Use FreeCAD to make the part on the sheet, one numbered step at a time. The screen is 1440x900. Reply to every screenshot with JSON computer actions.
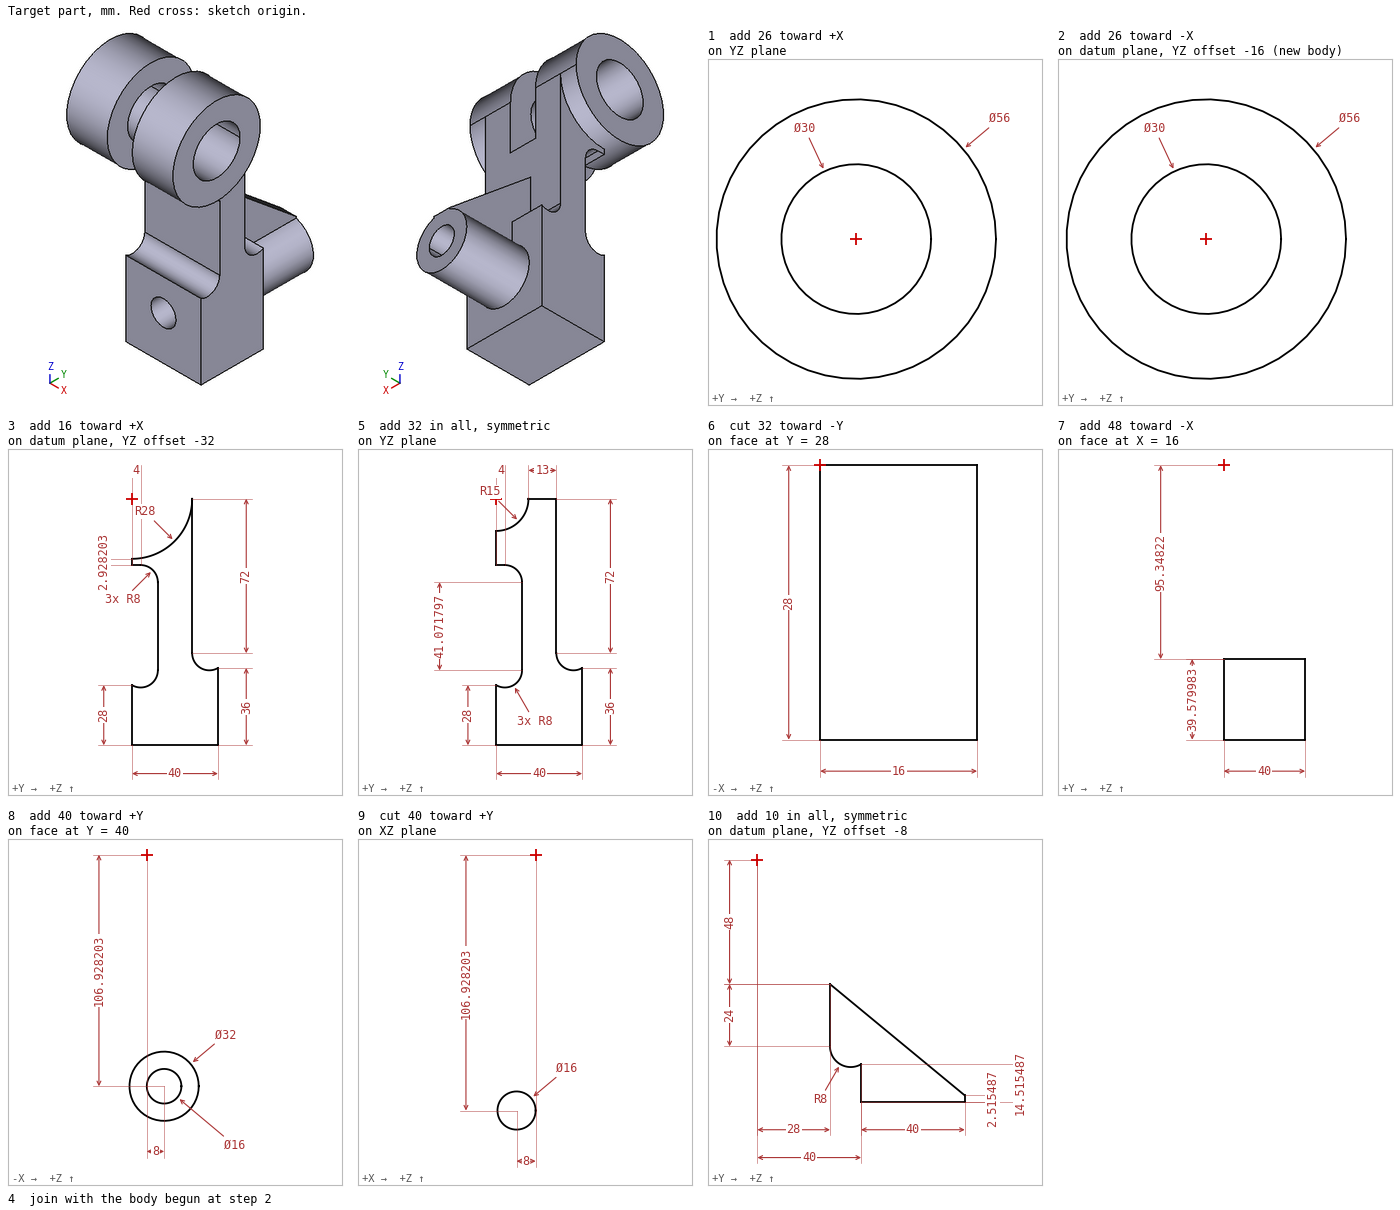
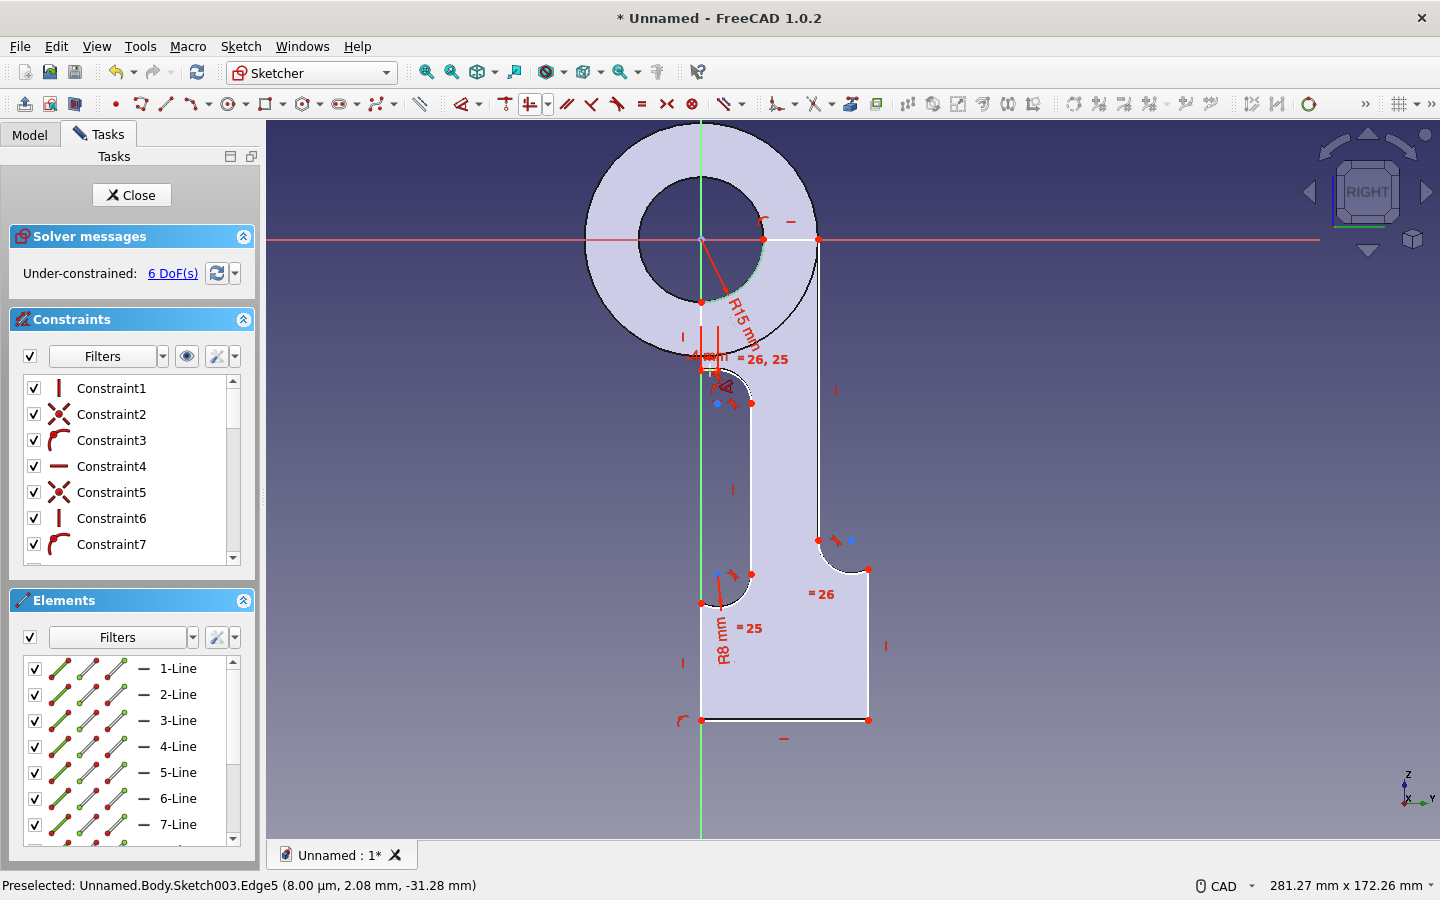
{"action": "left_click", "coordinate": [868, 615]}
{"action": "left_click", "coordinate": [902, 645]}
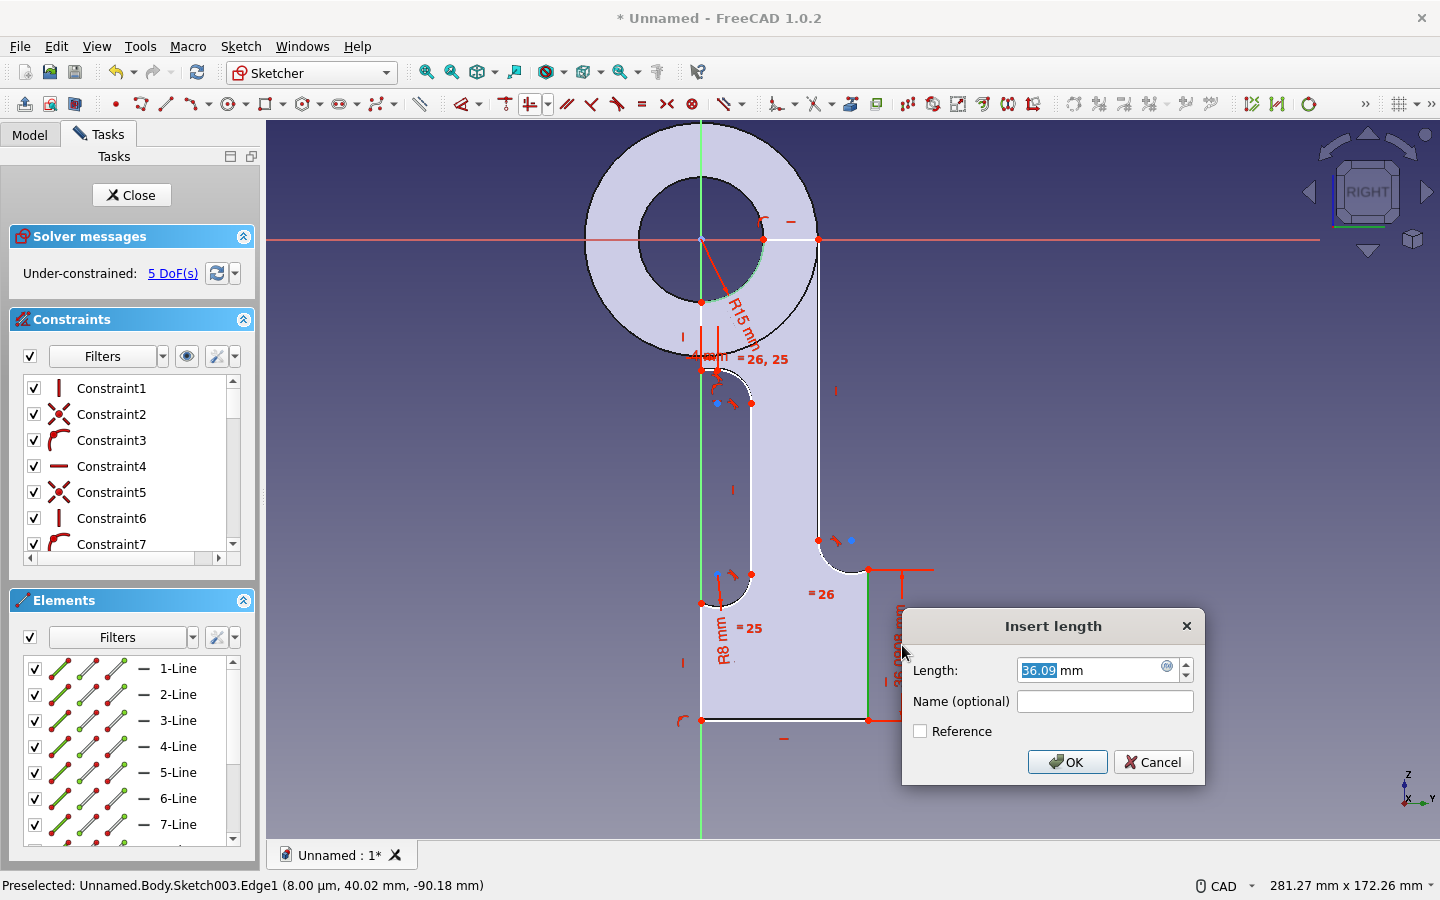
{"action": "type", "text": "36"}
{"action": "key", "text": "Return"}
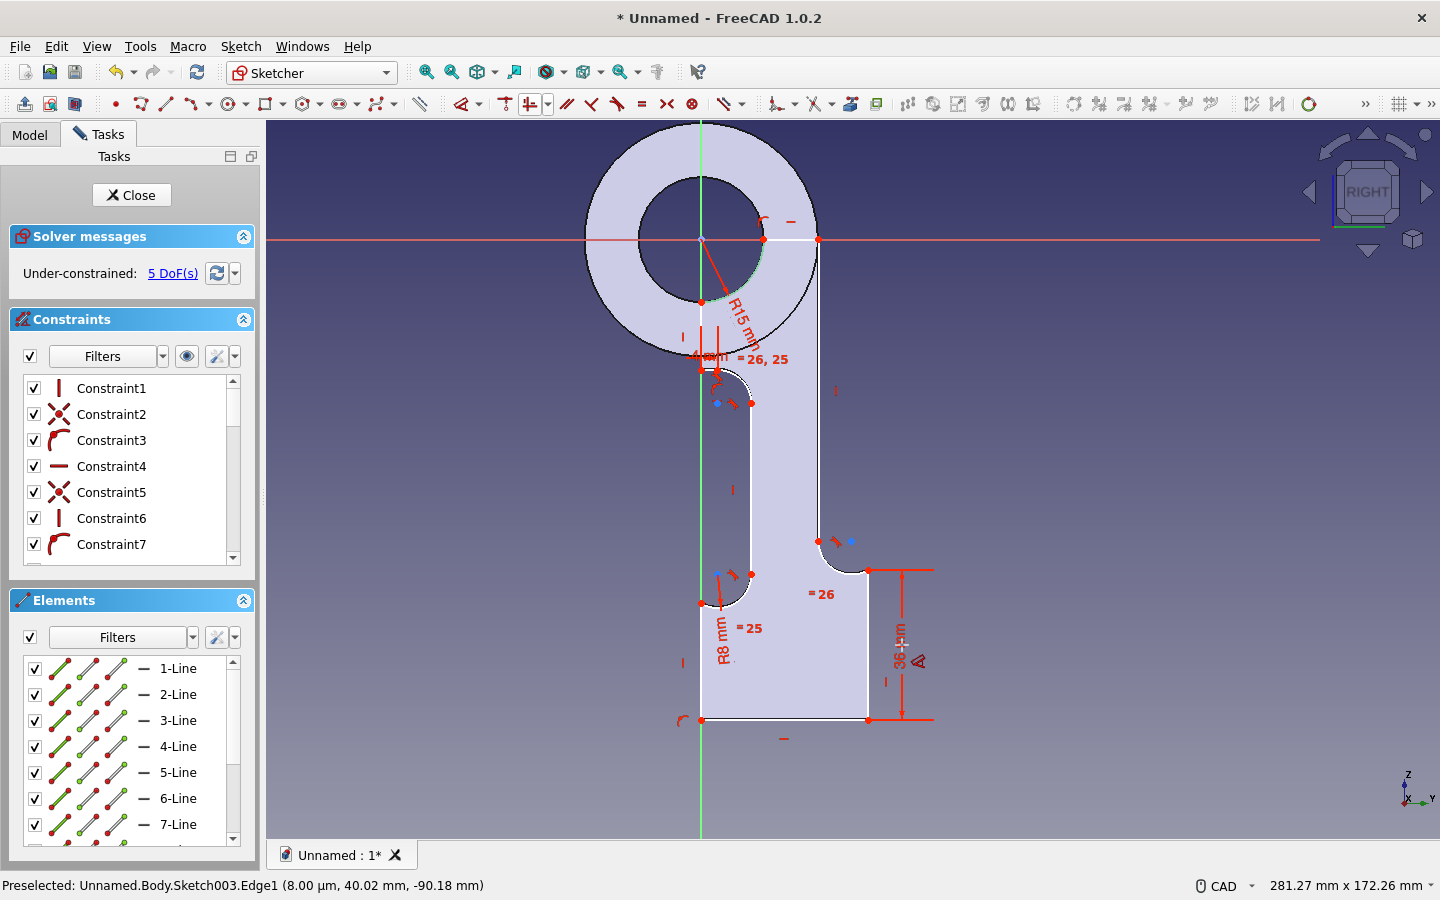
{"action": "left_click", "coordinate": [818, 720]}
{"action": "left_click", "coordinate": [785, 754]}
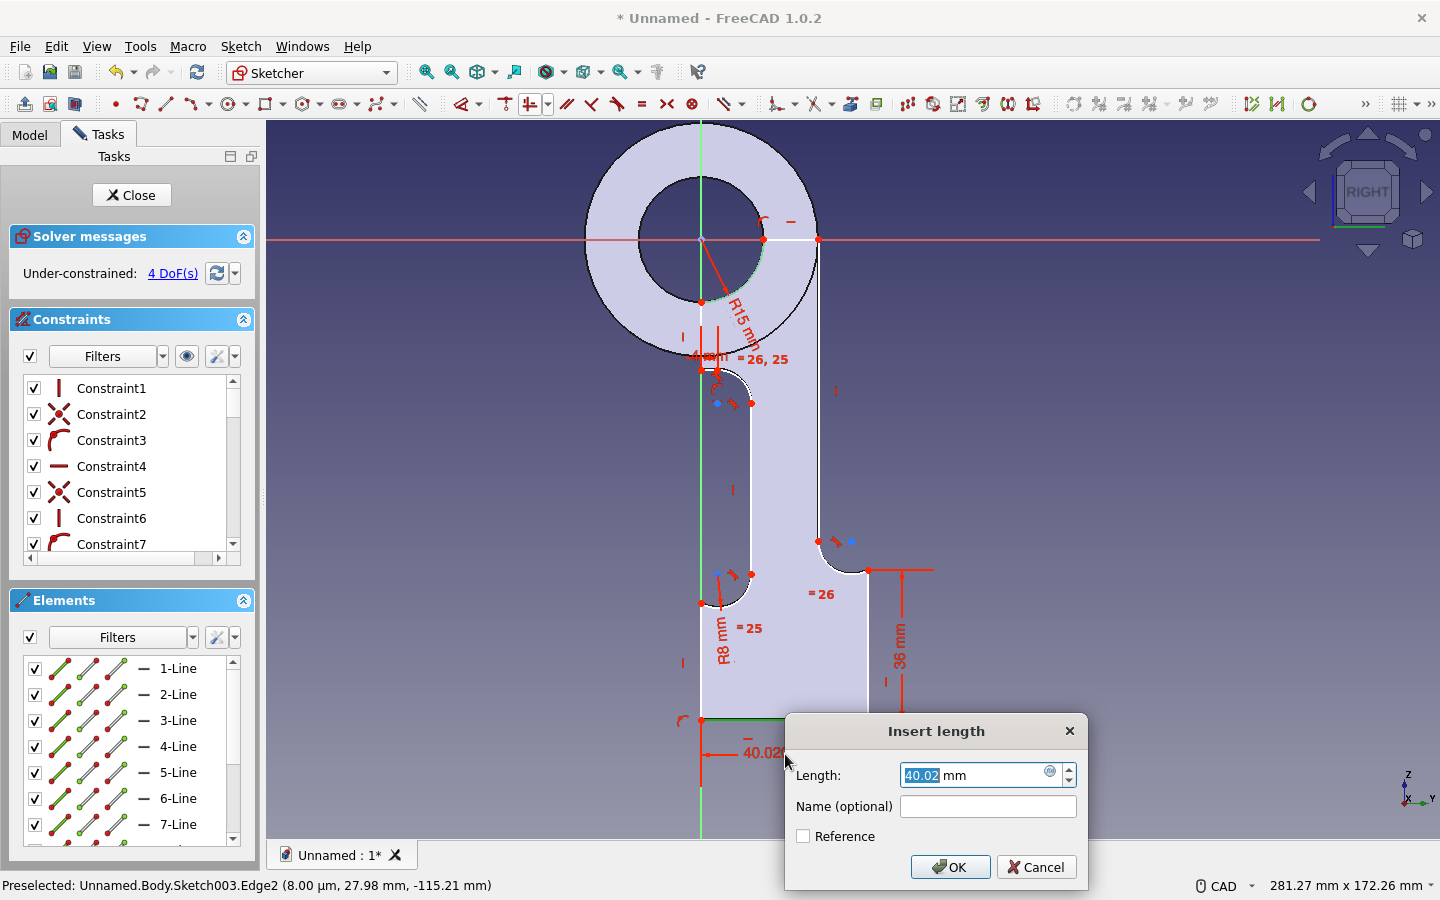
{"action": "type", "text": "40"}
{"action": "key", "text": "Return"}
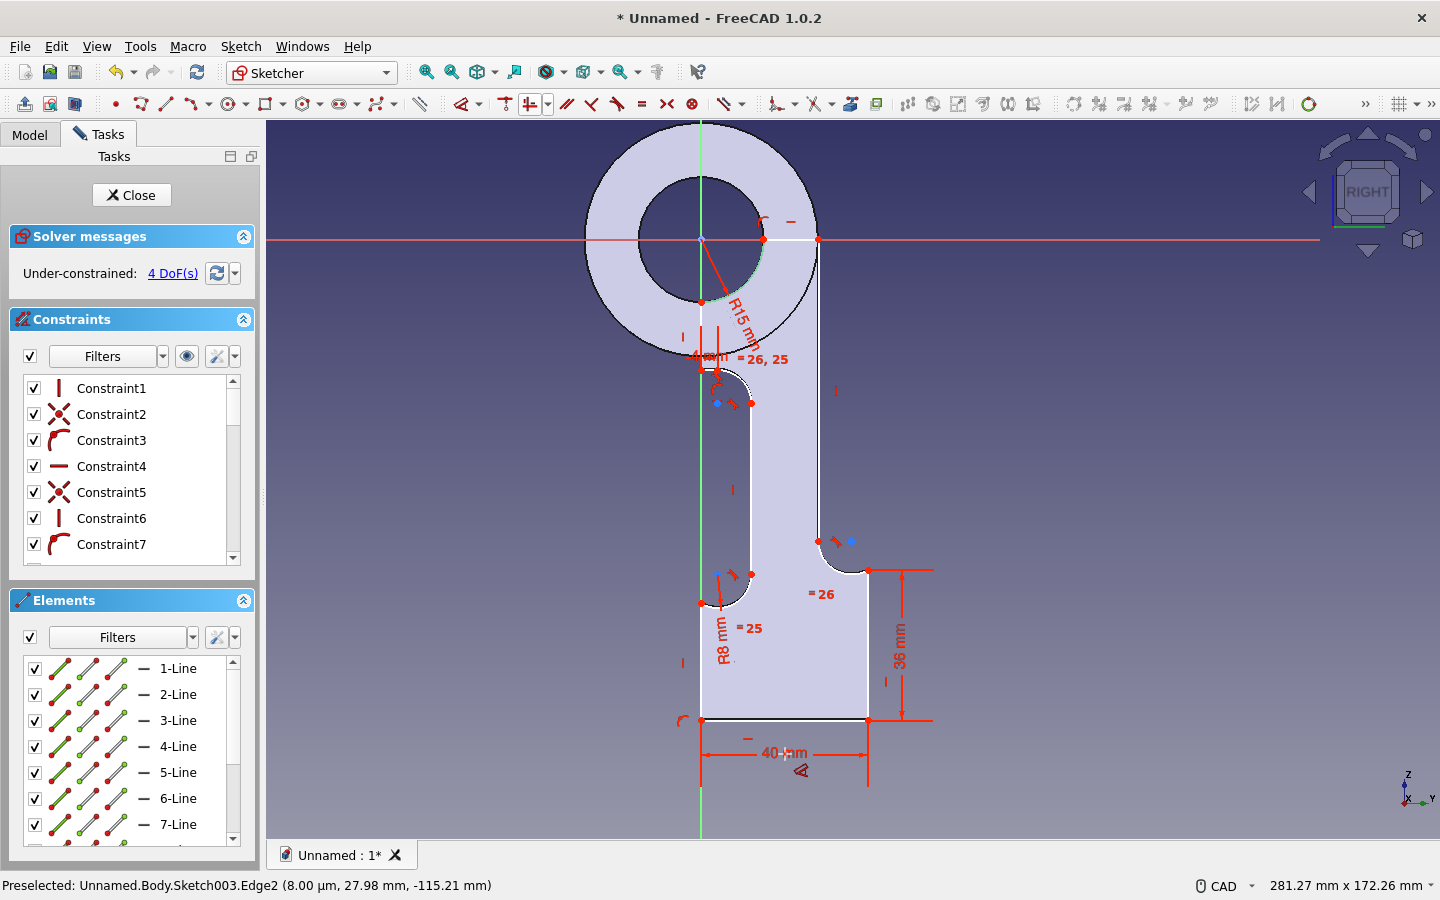
{"action": "left_click", "coordinate": [701, 685]}
{"action": "left_click", "coordinate": [667, 662]}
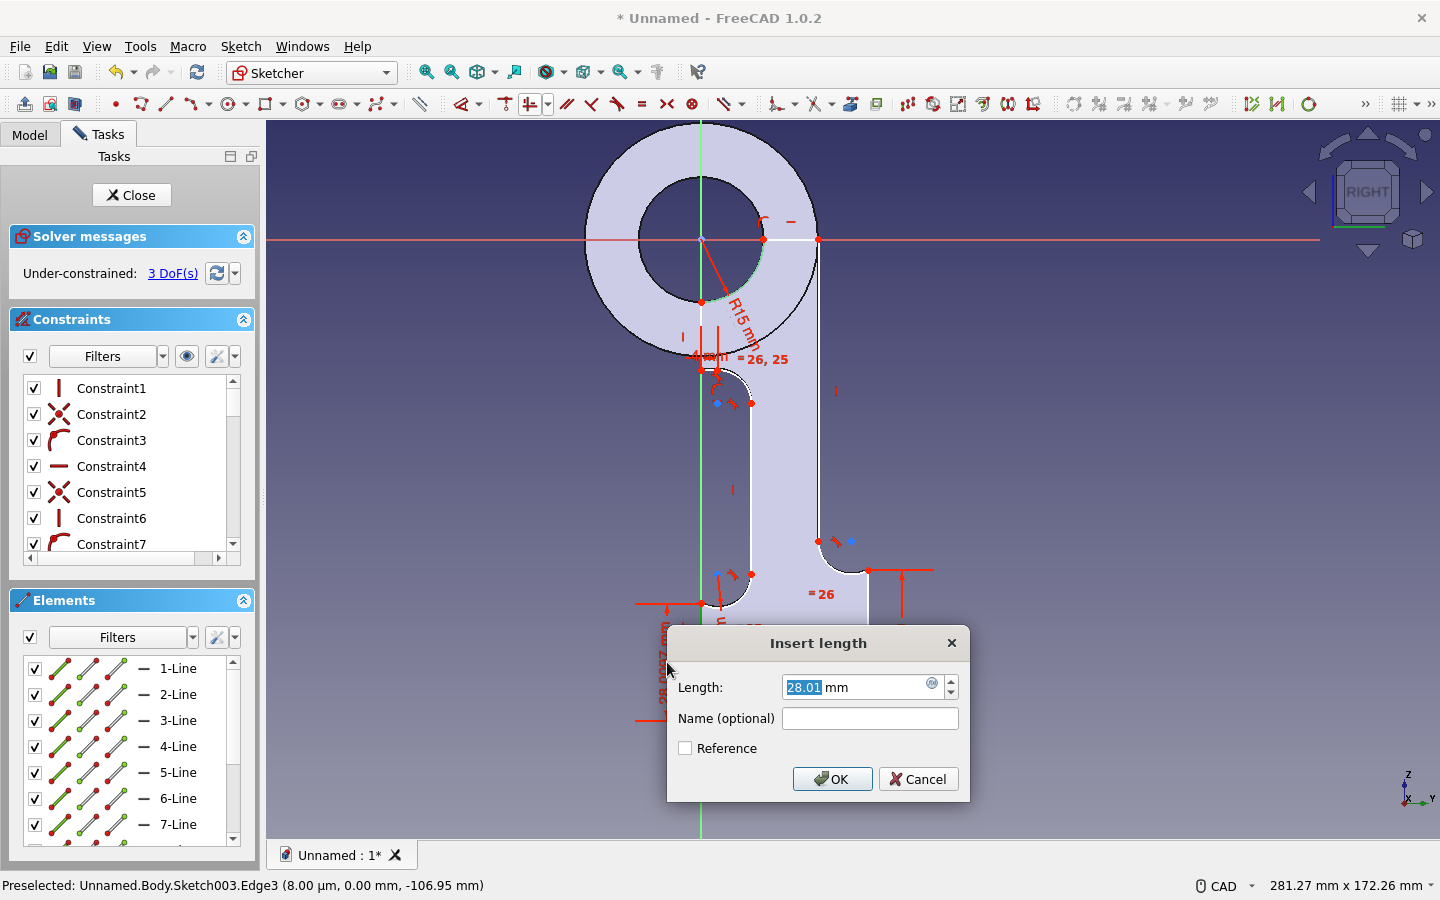
{"action": "type", "text": "28"}
{"action": "key", "text": "Return"}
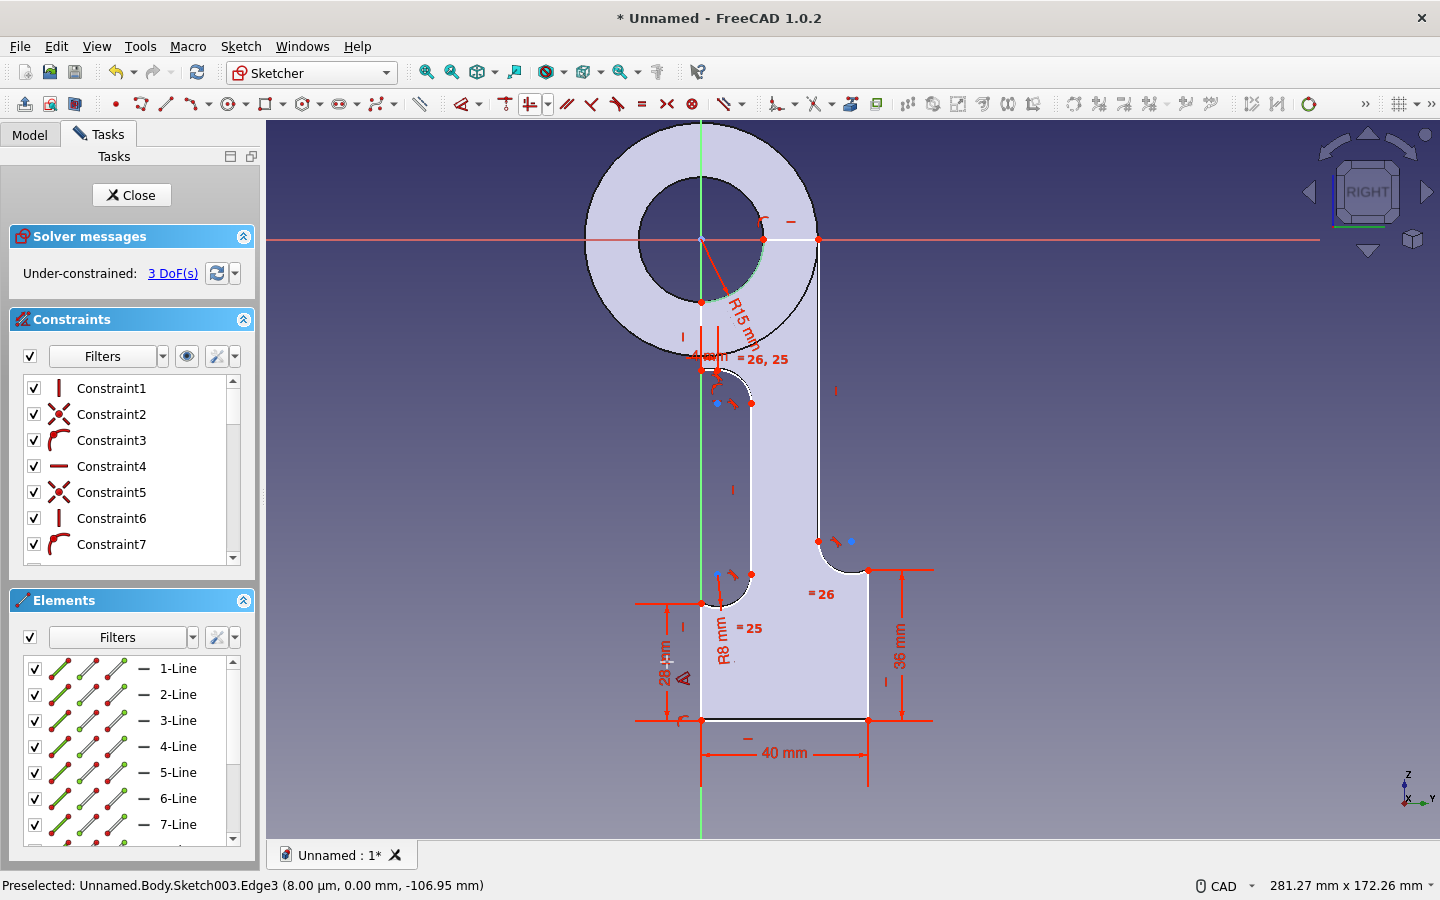
{"action": "left_click", "coordinate": [780, 240]}
{"action": "left_click", "coordinate": [791, 206]}